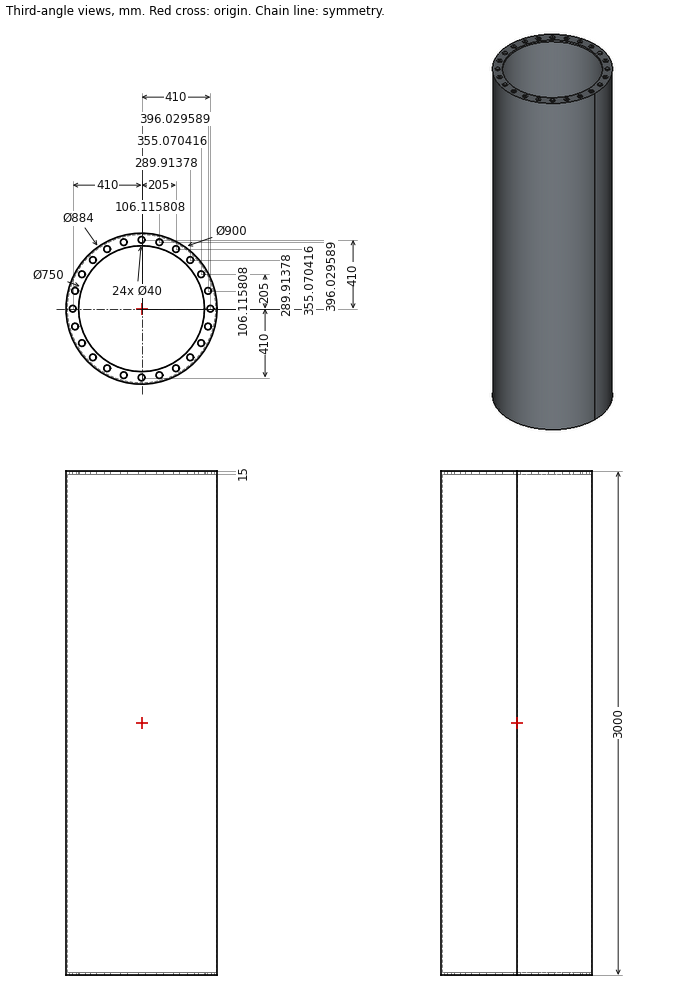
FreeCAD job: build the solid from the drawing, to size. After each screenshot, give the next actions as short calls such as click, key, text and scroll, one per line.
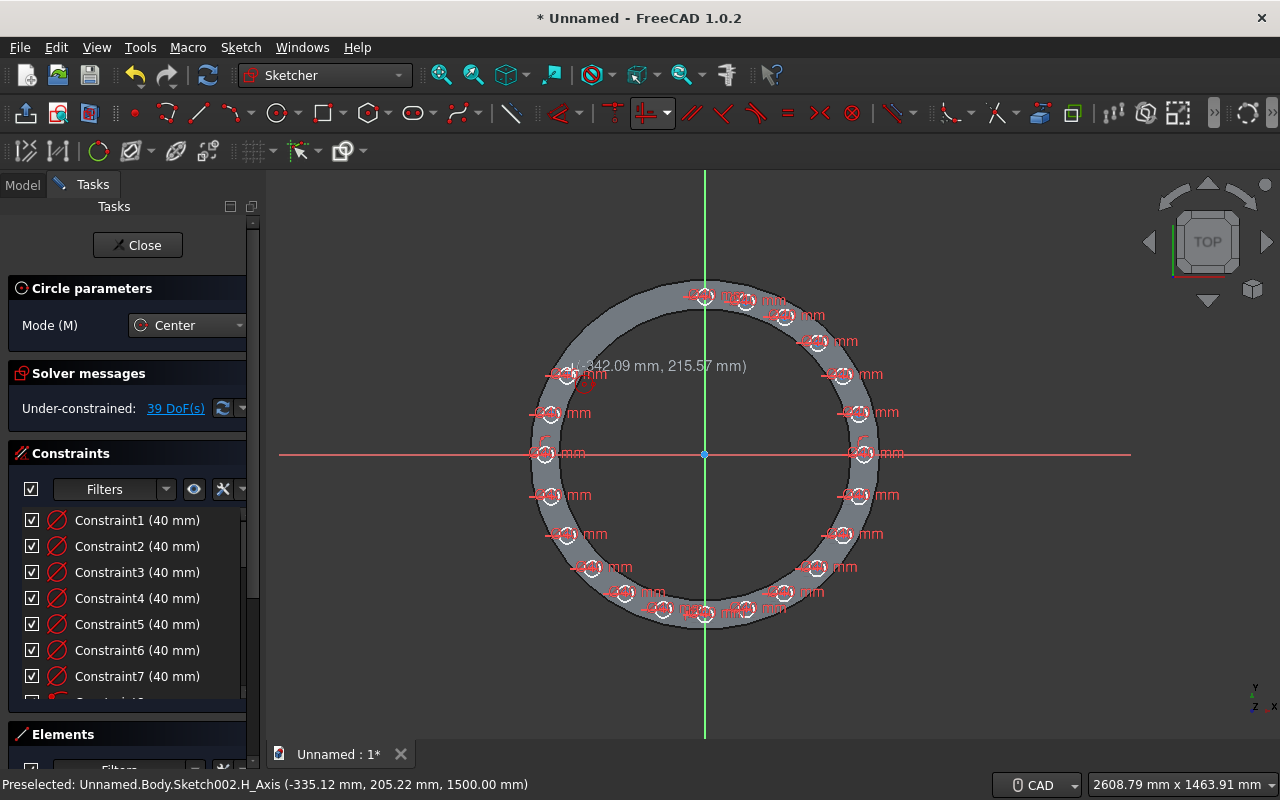
scroll(592, 342, up, 6)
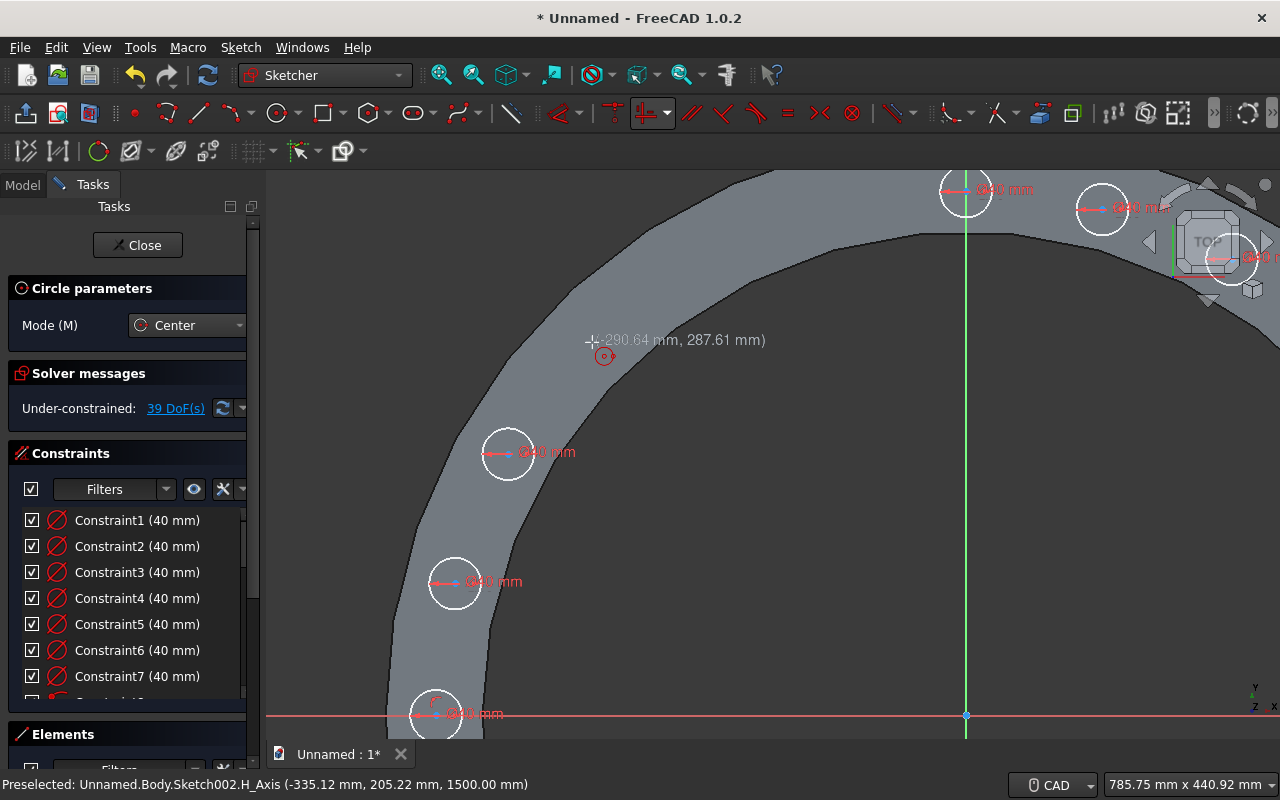
scroll(592, 342, down, 6)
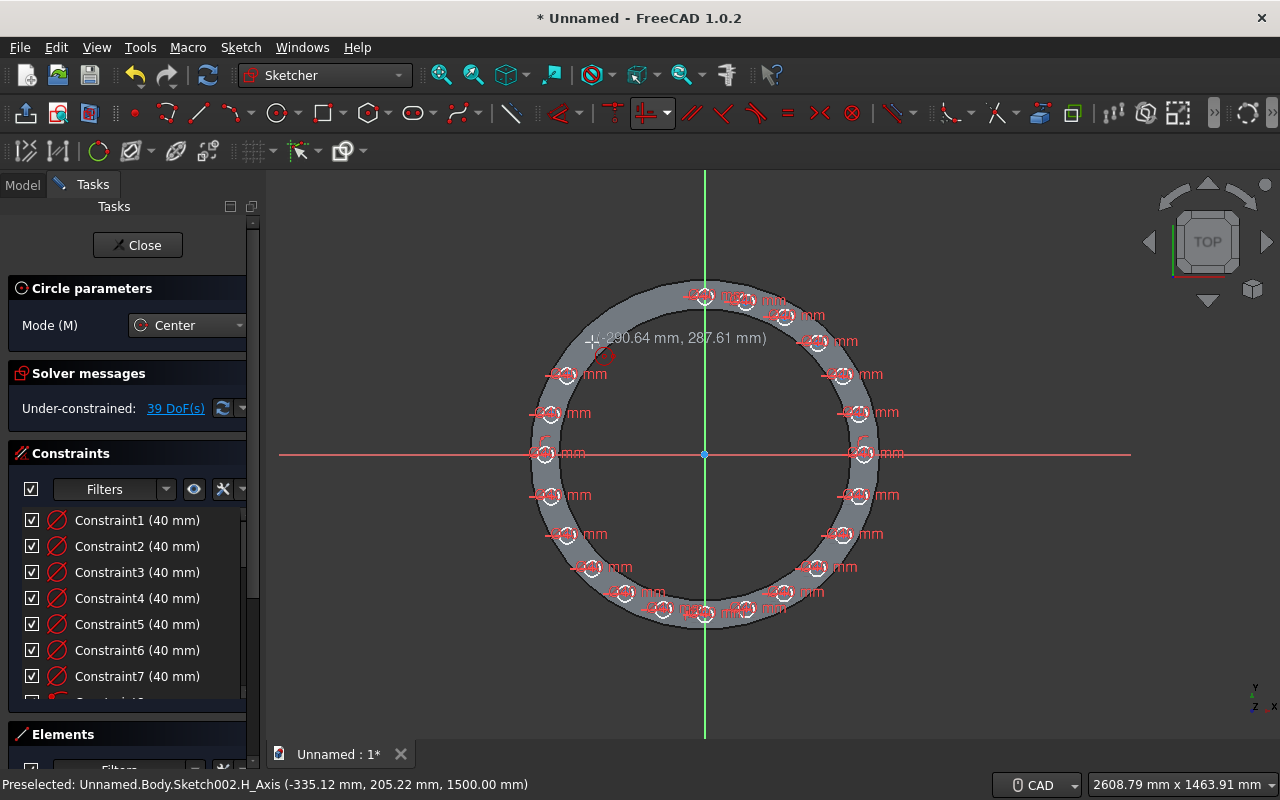
click(592, 342)
move(598, 337)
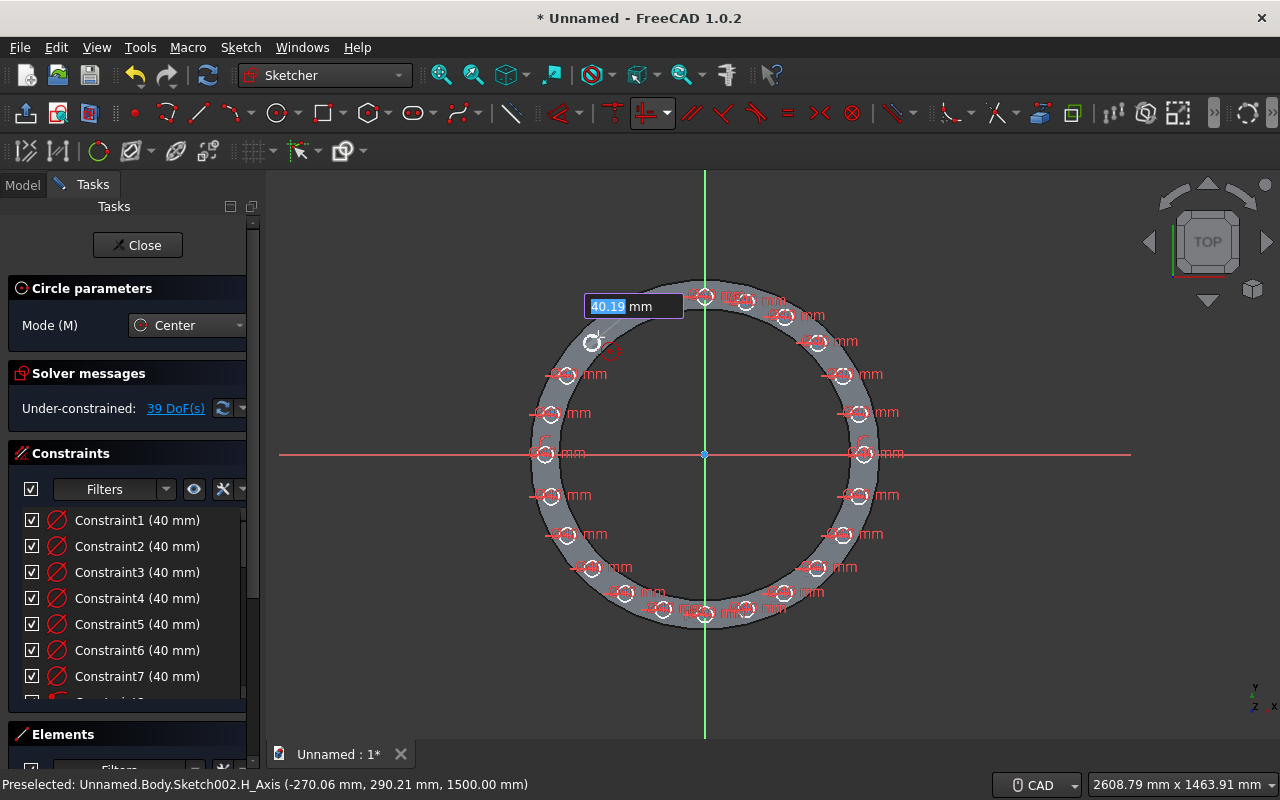
text(40)
key(Return)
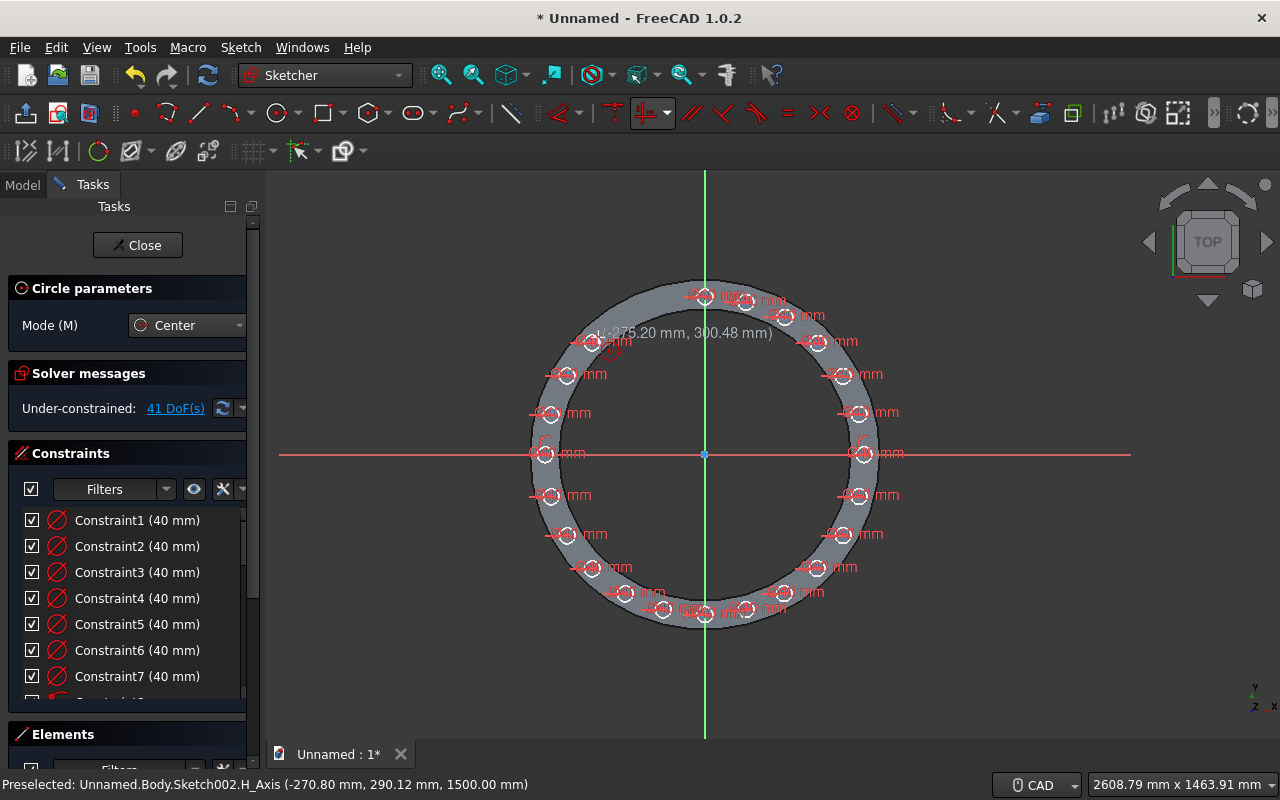
scroll(625, 317, up, 6)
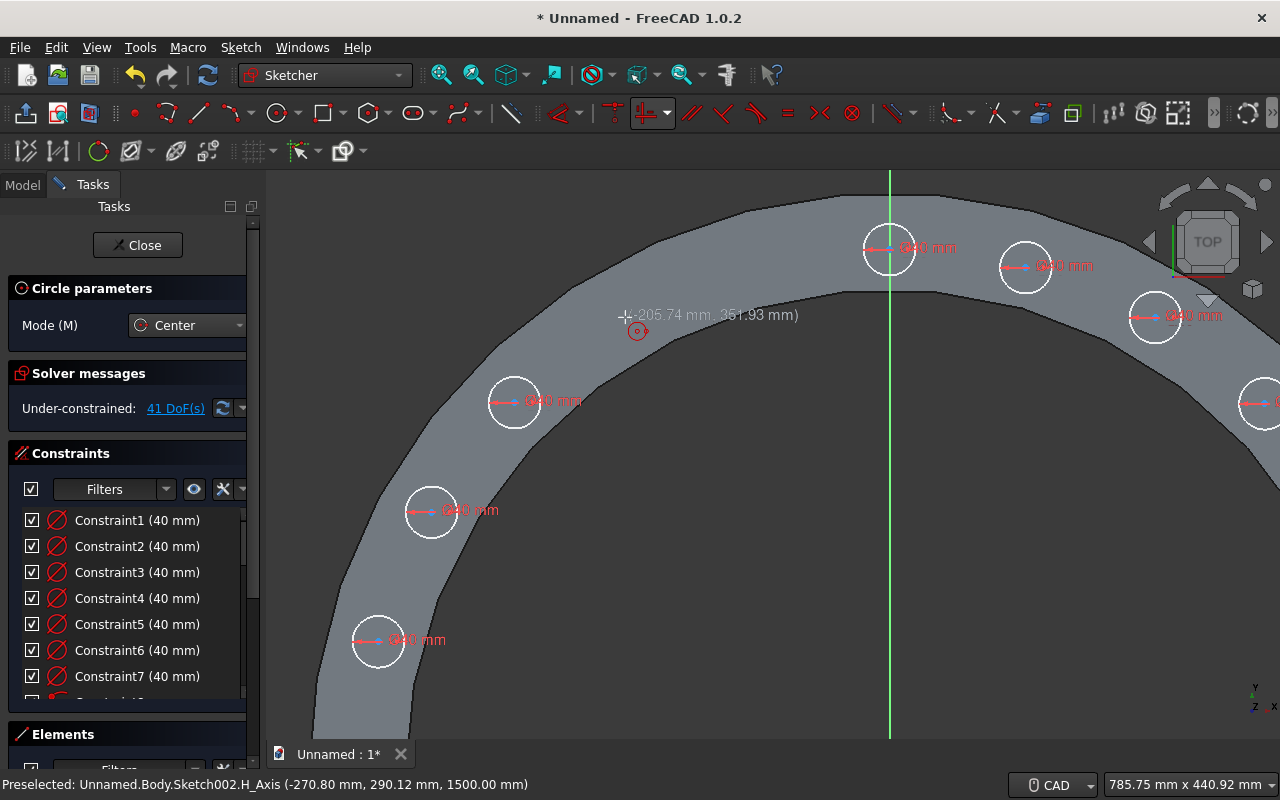
scroll(625, 317, down, 6)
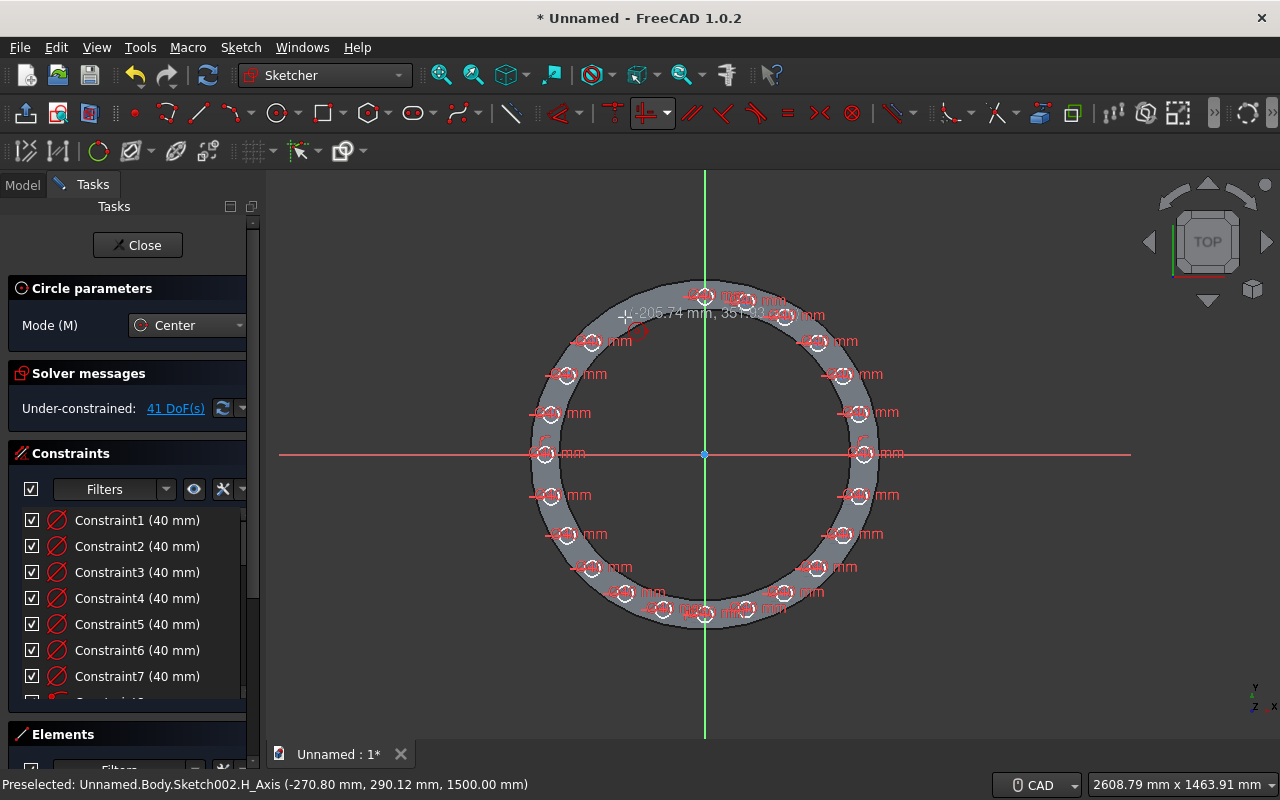
click(625, 317)
move(631, 311)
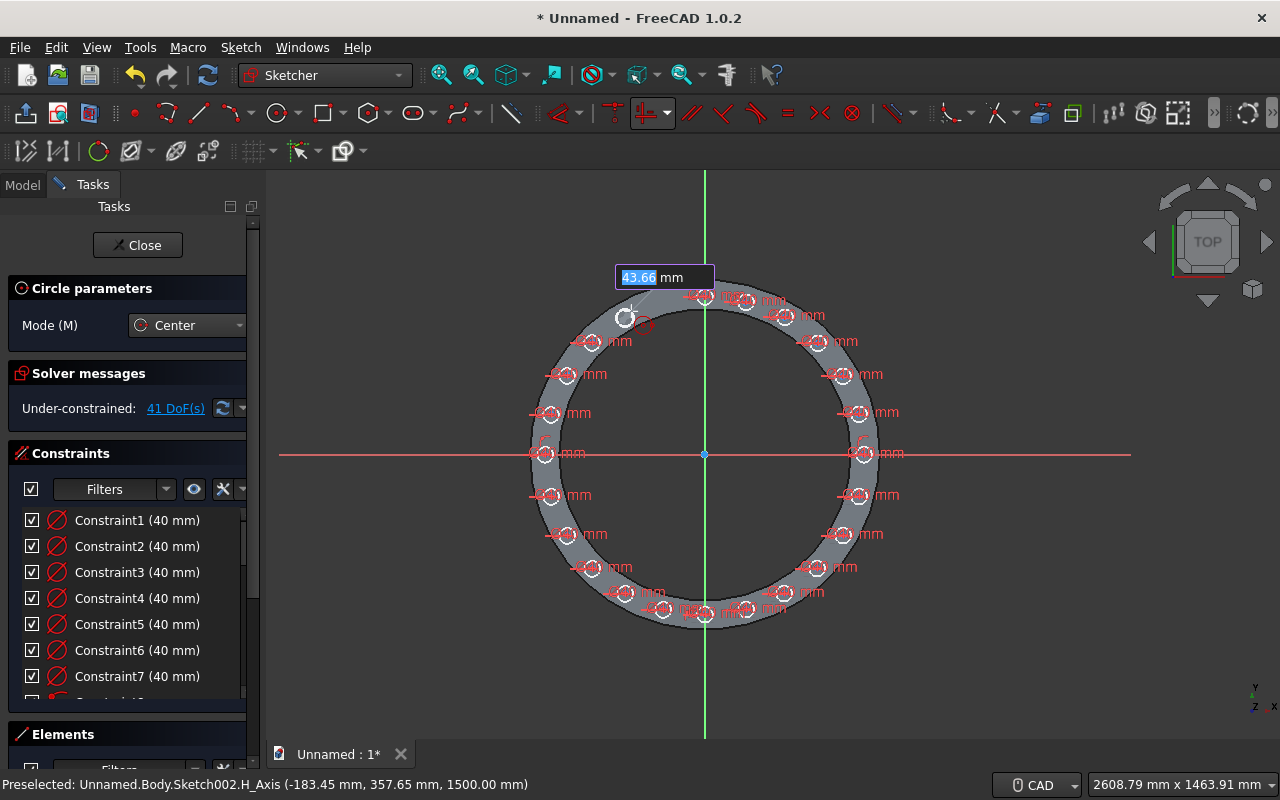
text(40)
key(Return)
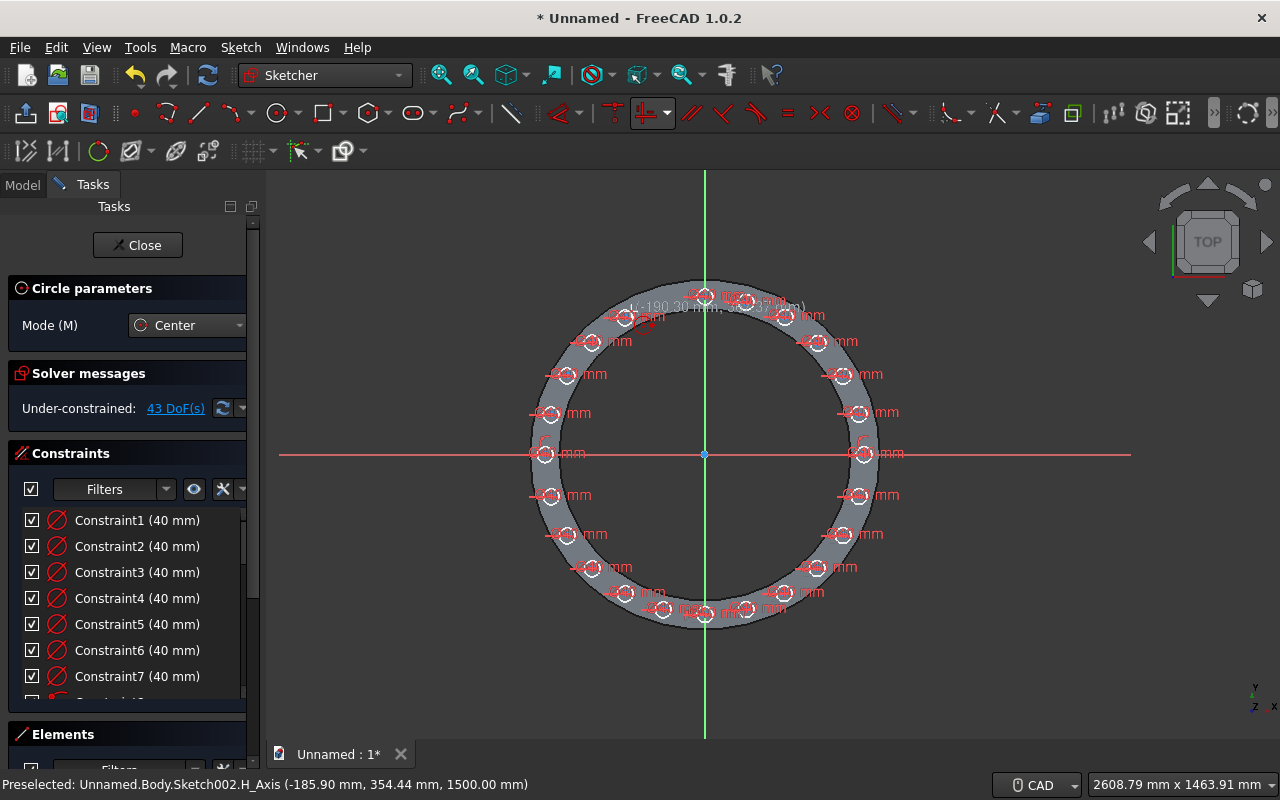
scroll(664, 301, up, 6)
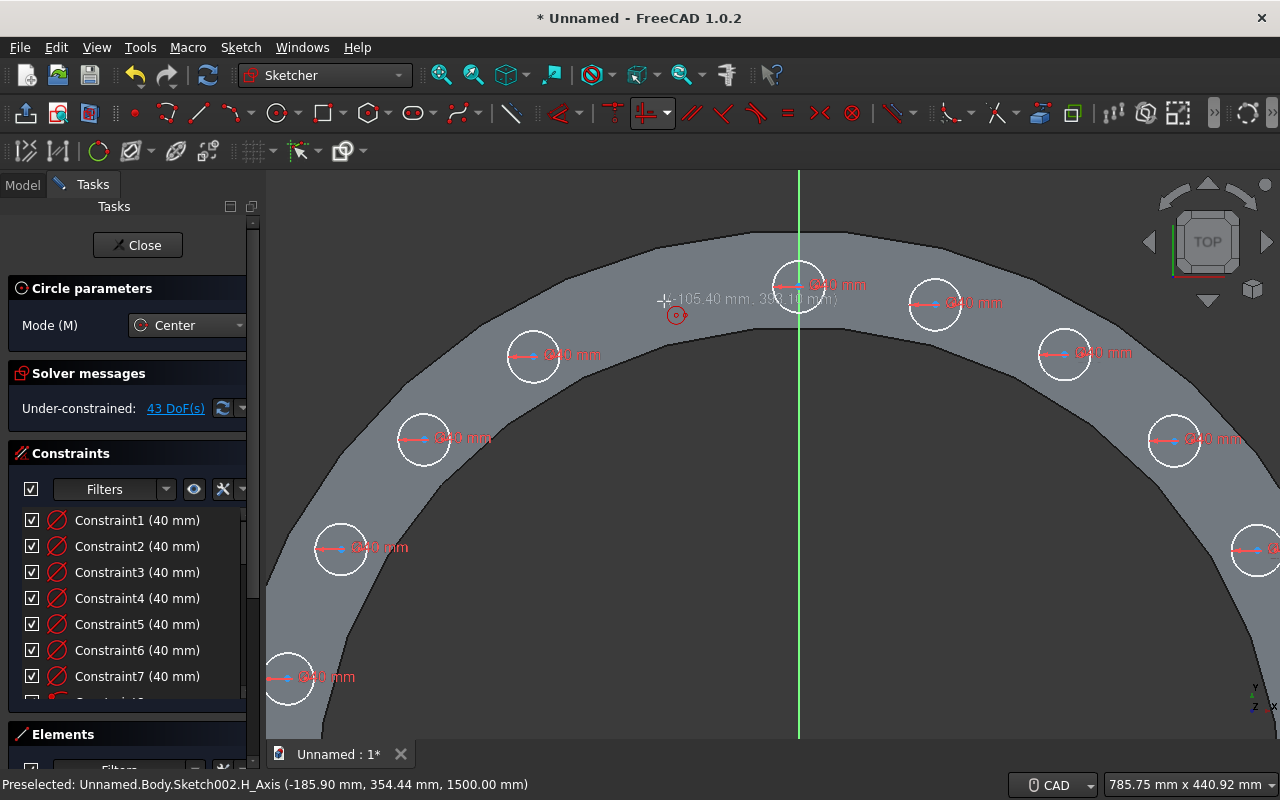
scroll(664, 301, down, 6)